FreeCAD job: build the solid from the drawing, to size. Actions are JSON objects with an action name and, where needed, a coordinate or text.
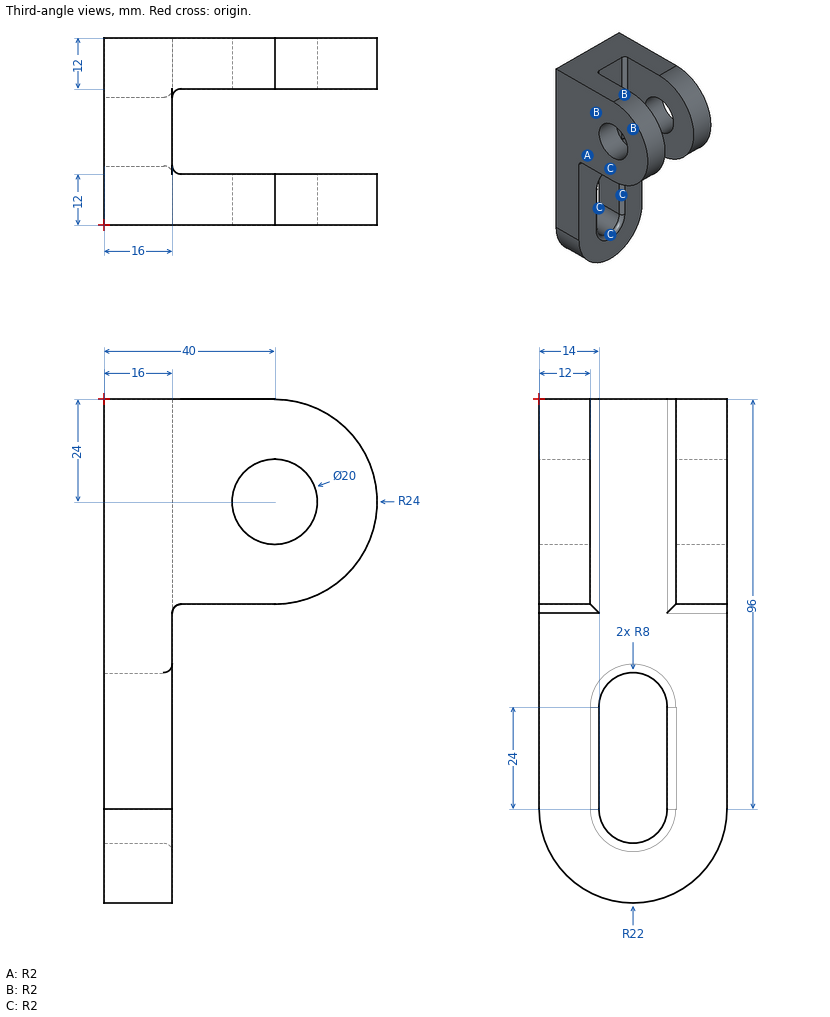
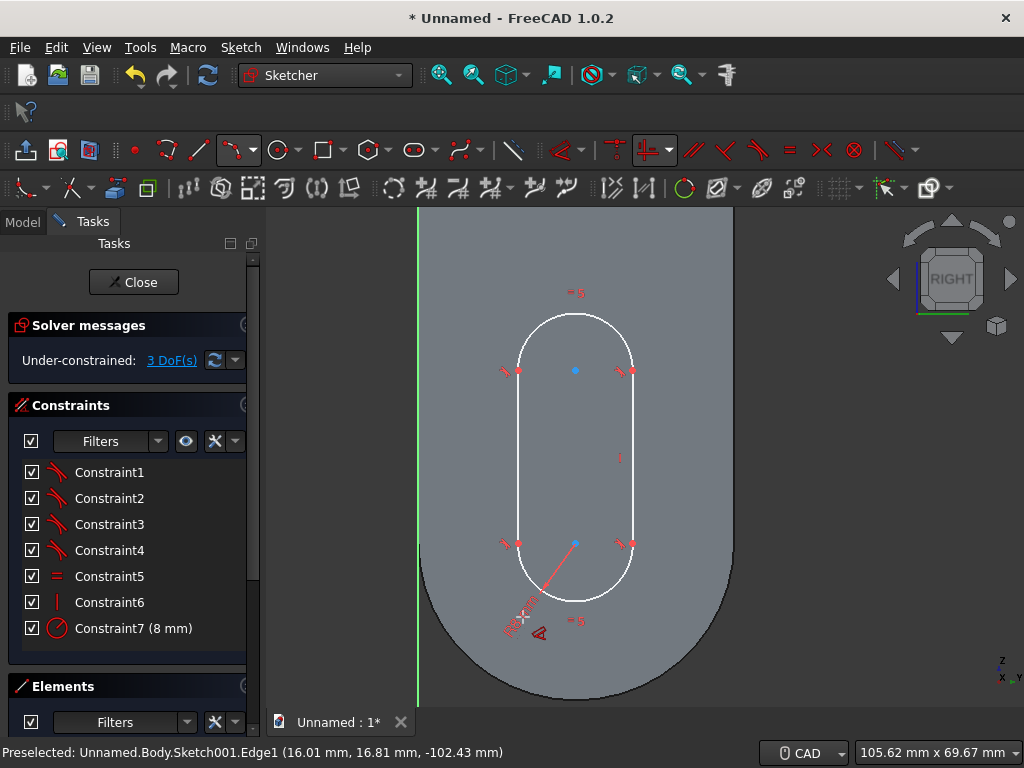
{"action": "left_click", "coordinate": [518, 492]}
{"action": "left_click", "coordinate": [484, 458]}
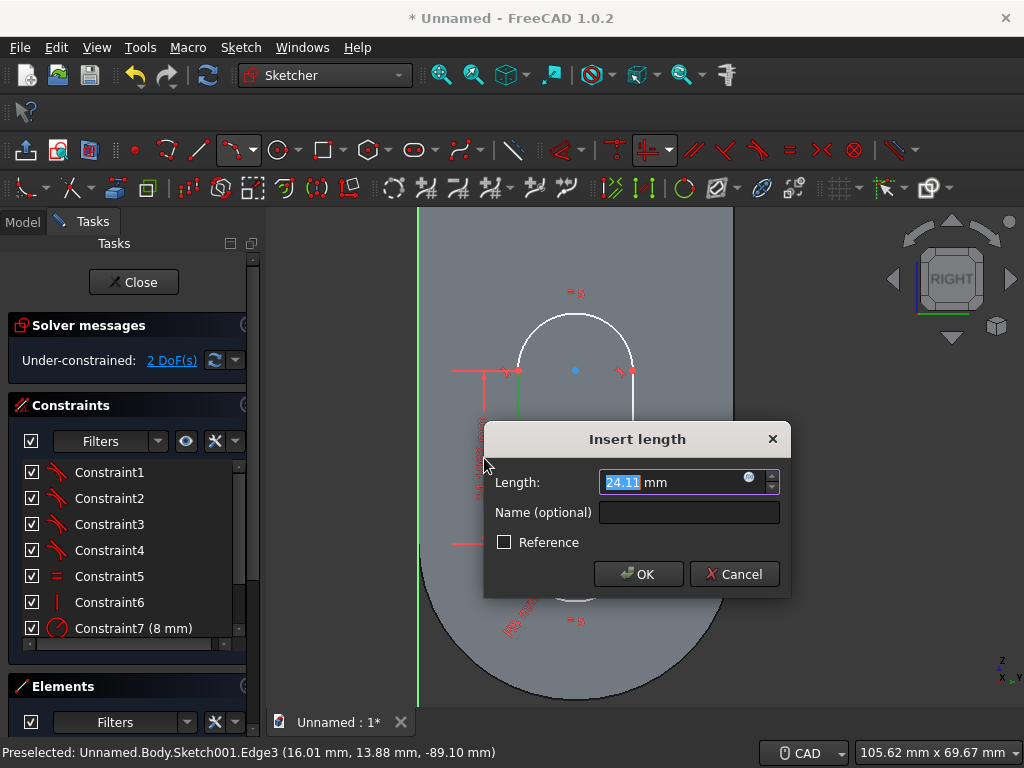
{"action": "type", "text": "24"}
{"action": "key", "text": "Return"}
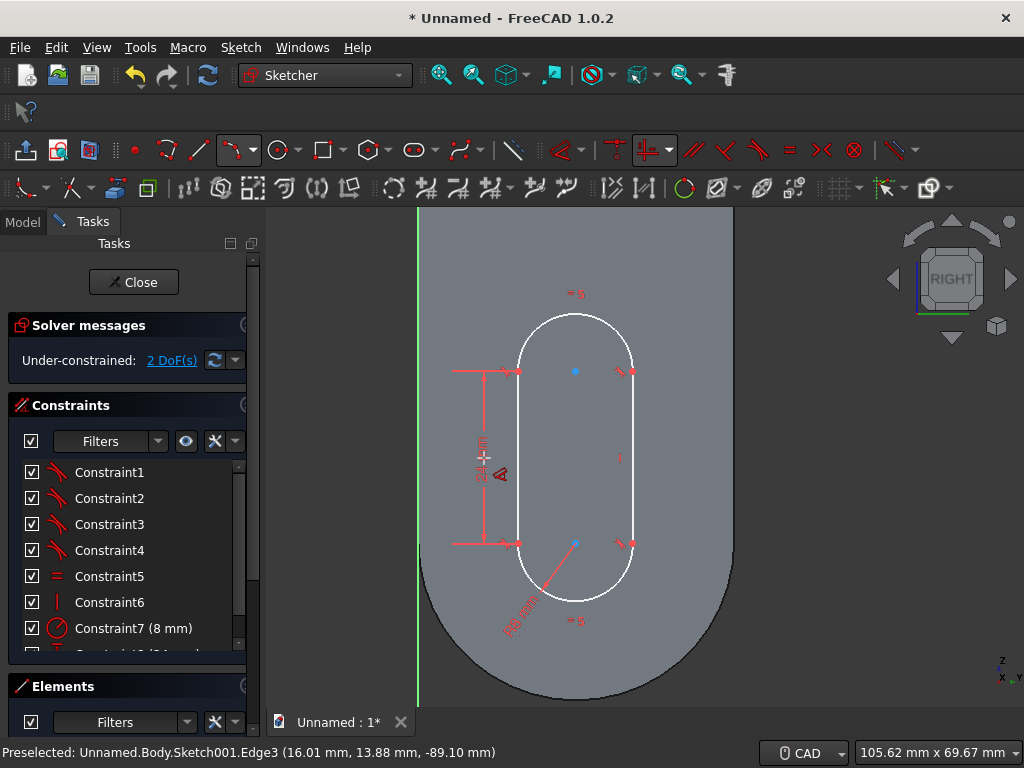
{"action": "left_click", "coordinate": [518, 544]}
{"action": "left_click", "coordinate": [468, 578]}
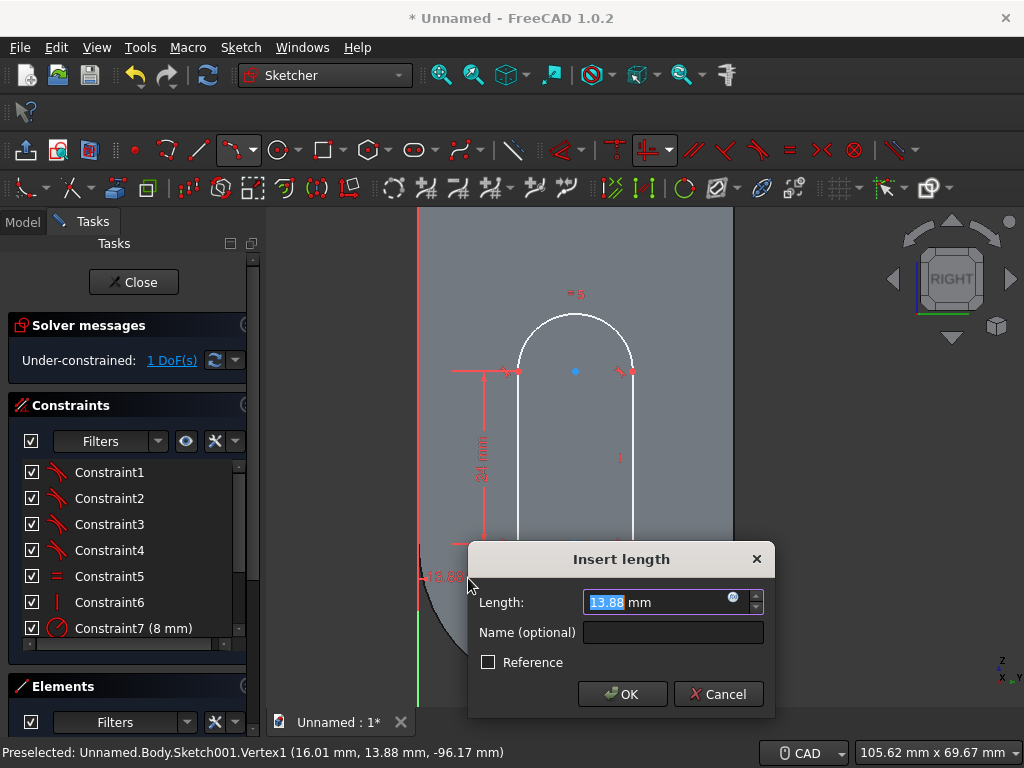
{"action": "type", "text": "14"}
{"action": "key", "text": "Return"}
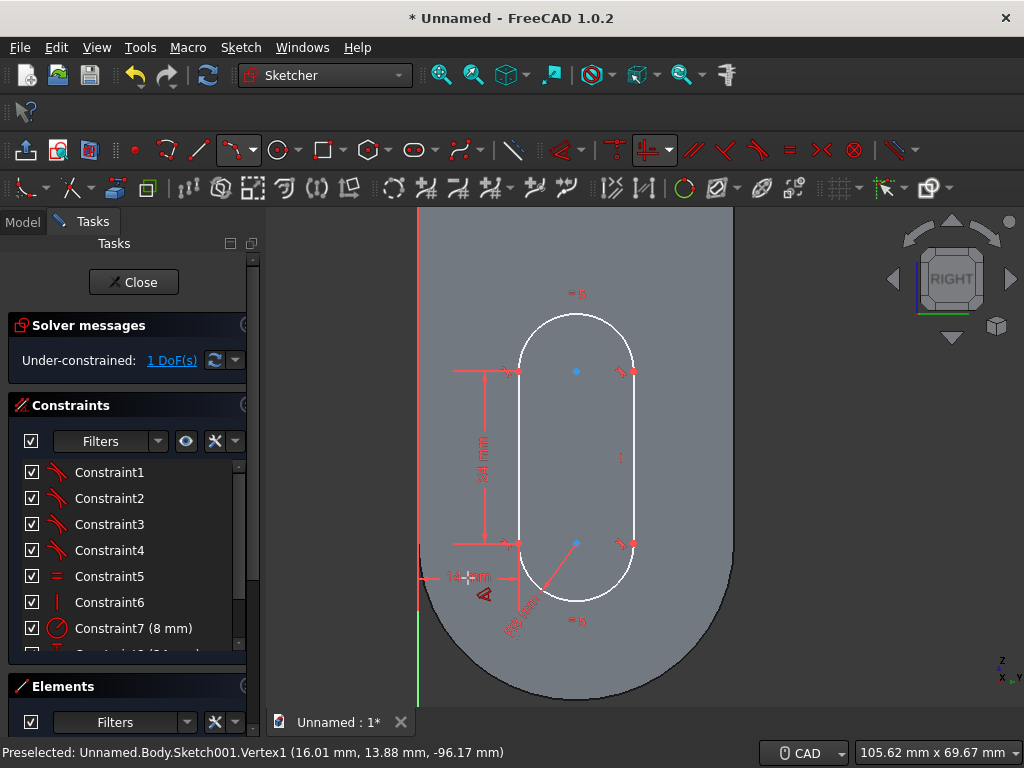
{"action": "left_click", "coordinate": [519, 544]}
{"action": "left_click", "coordinate": [384, 389]}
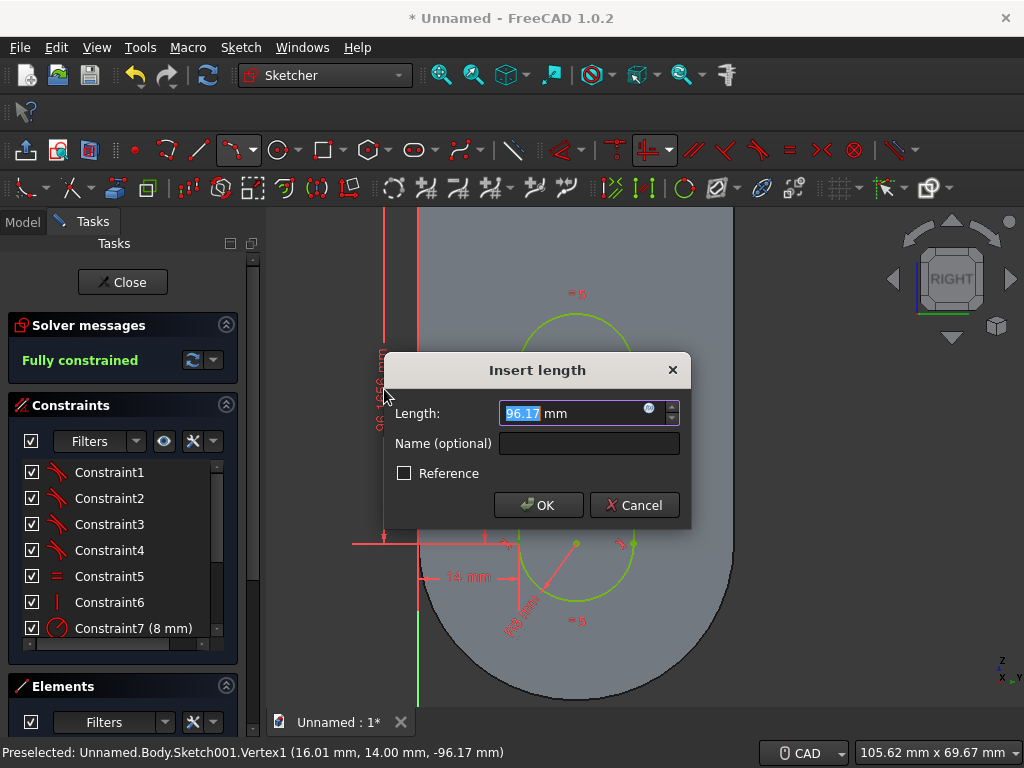
{"action": "type", "text": "96"}
{"action": "key", "text": "Return"}
{"action": "key", "text": "Escape"}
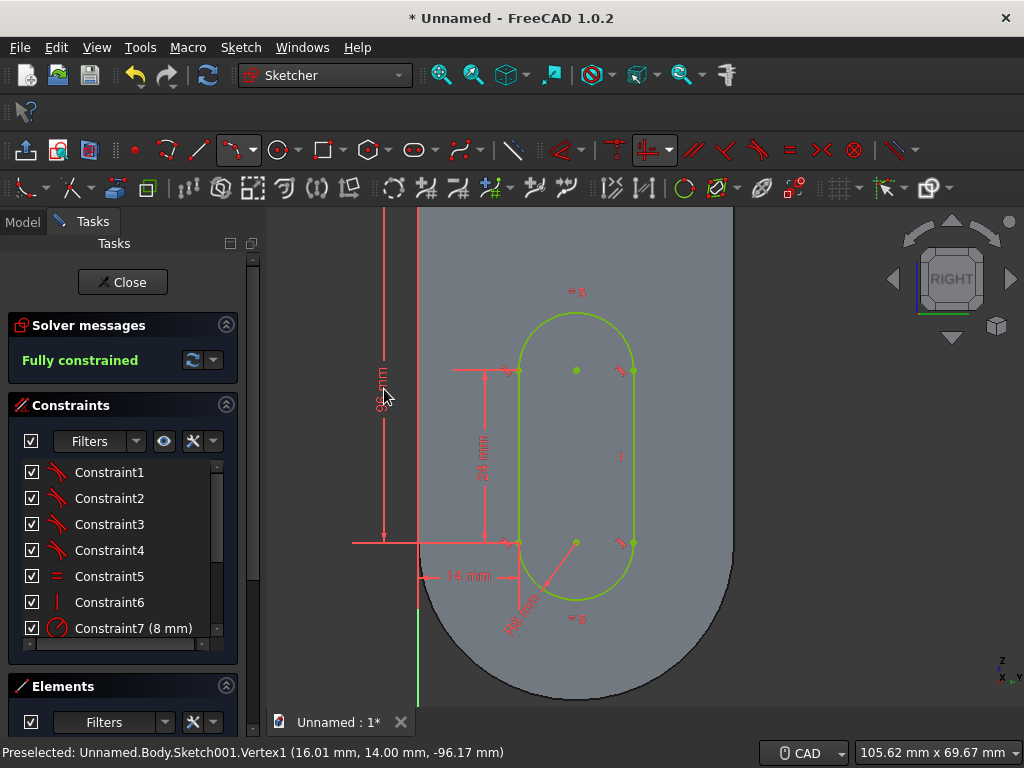
{"action": "left_click", "coordinate": [123, 282]}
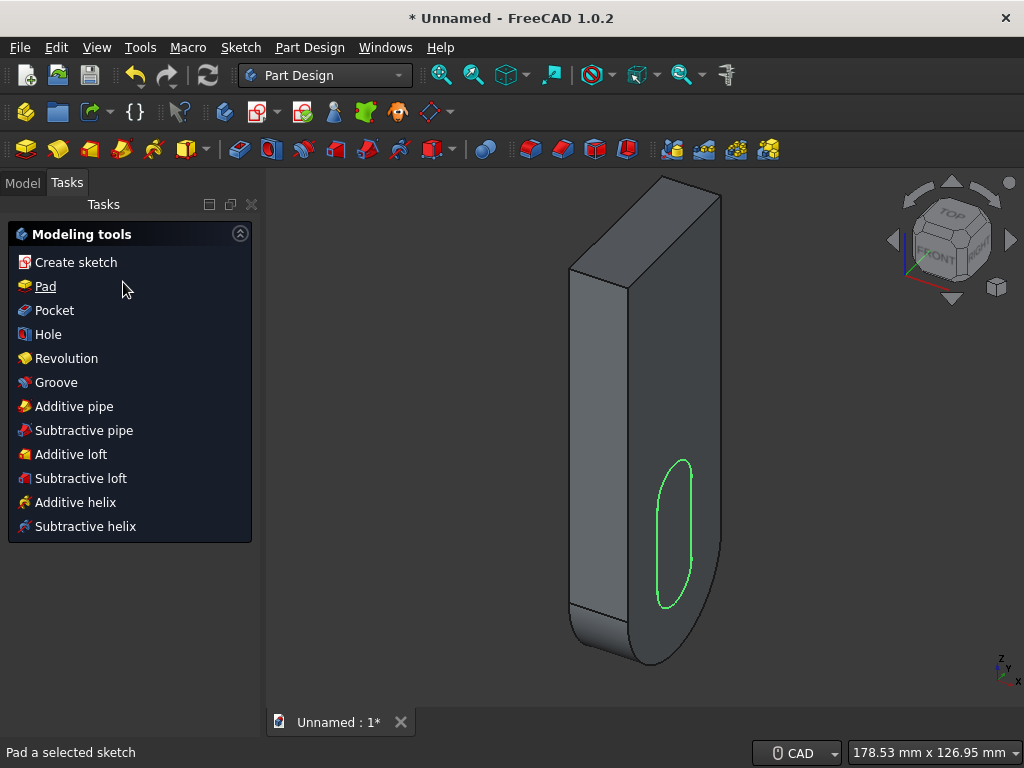
{"action": "left_click", "coordinate": [240, 150]}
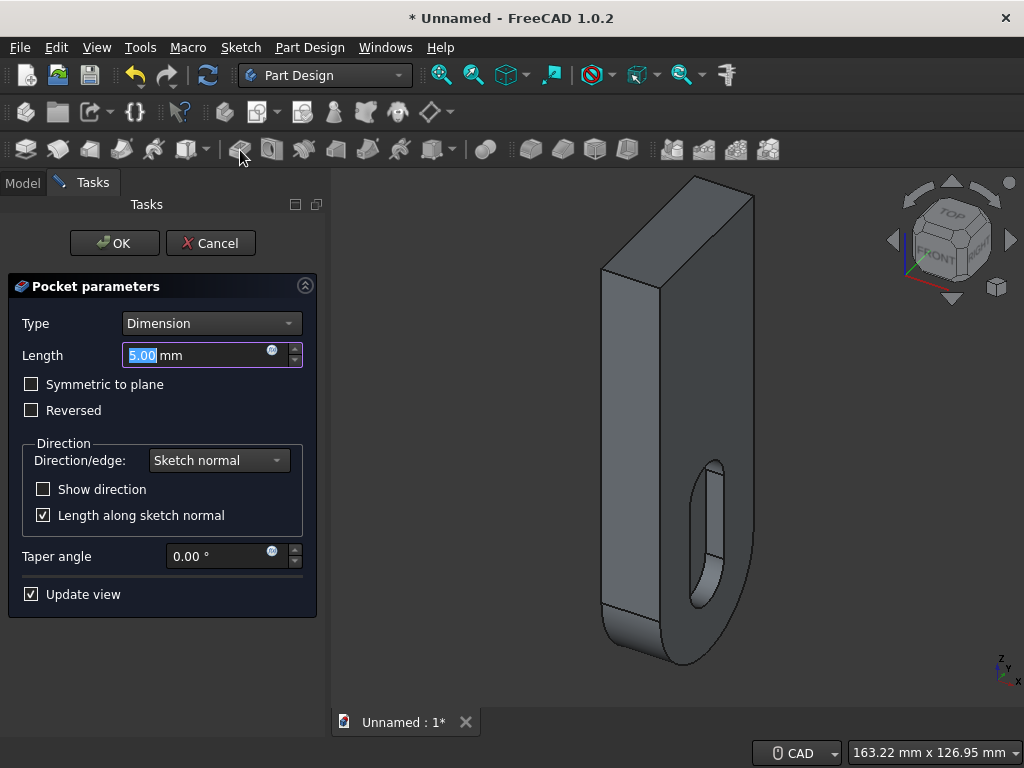
{"action": "type", "text": "16"}
{"action": "key", "text": "Tab"}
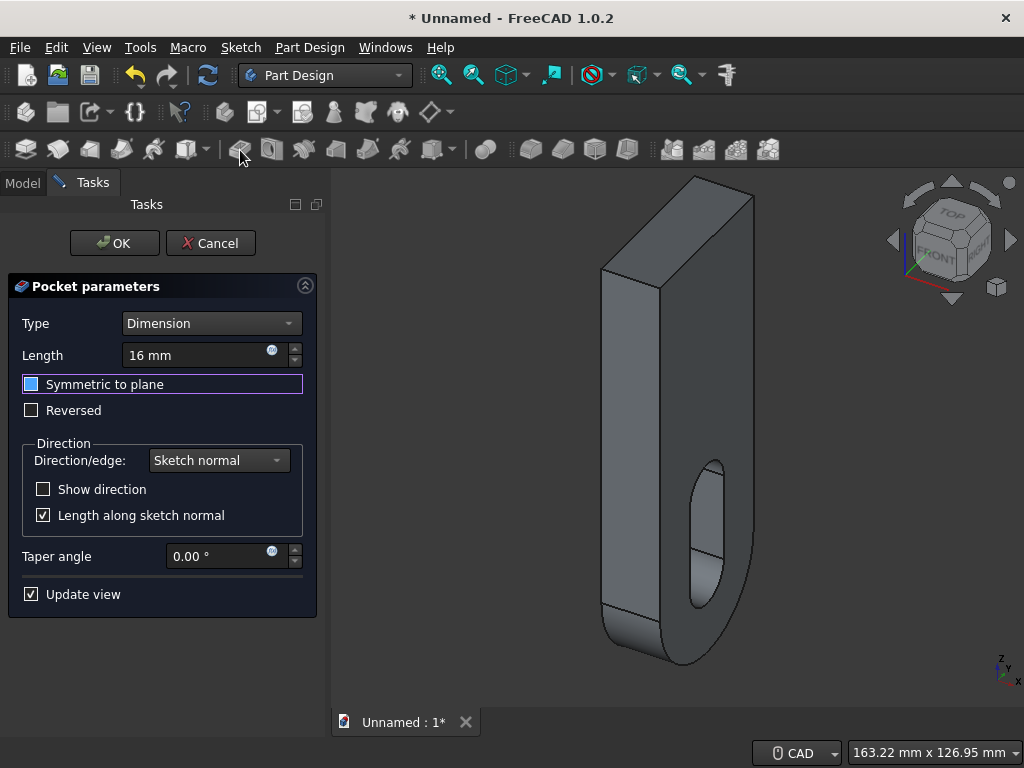
{"action": "left_click", "coordinate": [115, 243]}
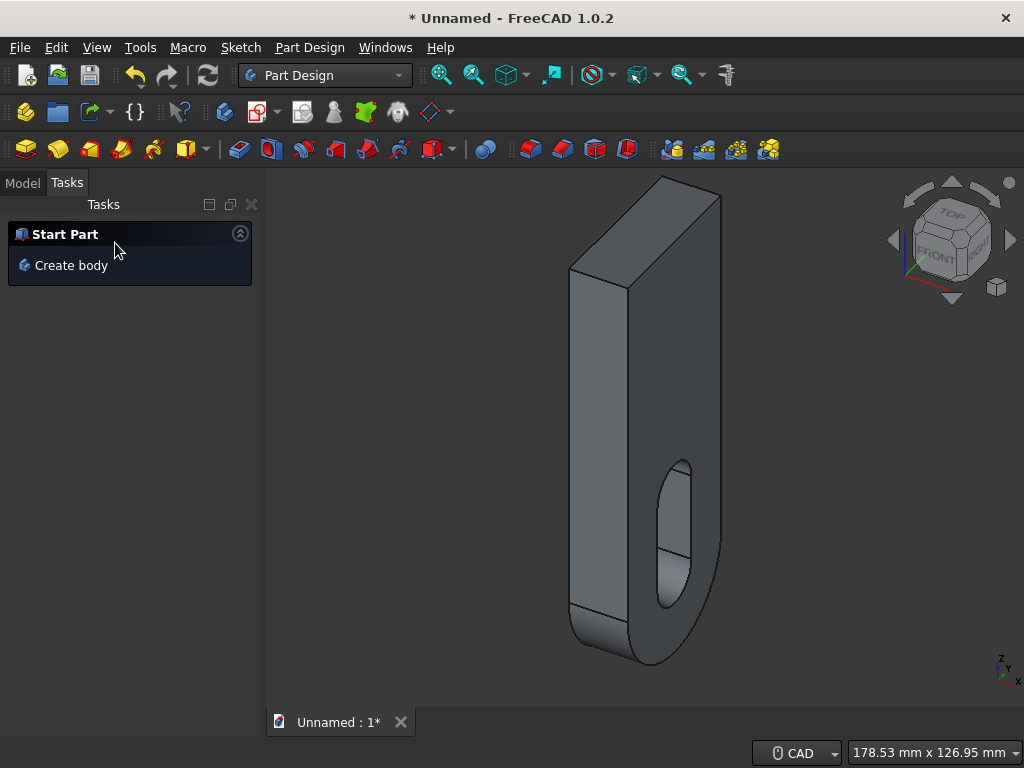
{"action": "left_click", "coordinate": [258, 112]}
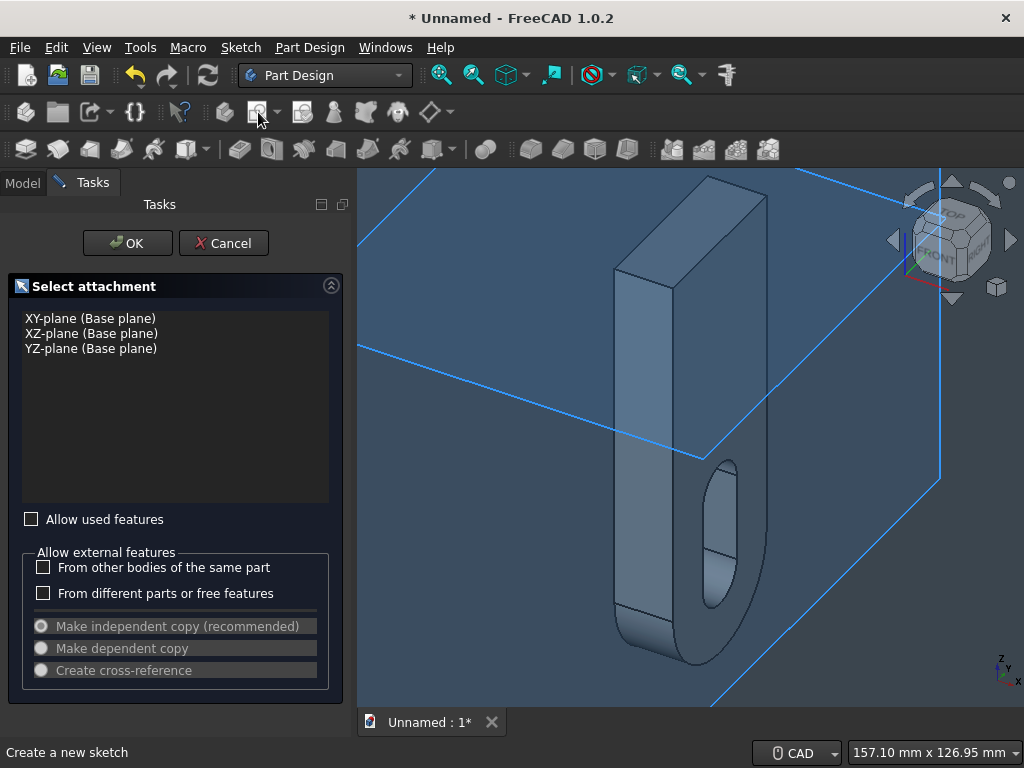
{"action": "left_click", "coordinate": [82, 334]}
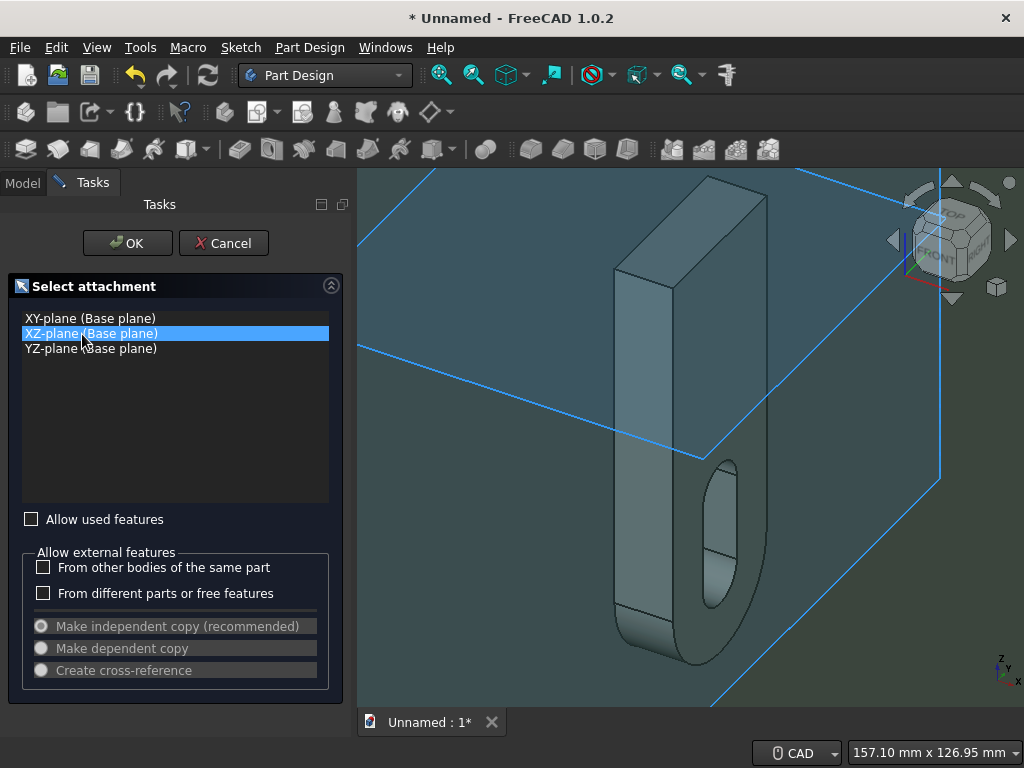
{"action": "left_click", "coordinate": [128, 243]}